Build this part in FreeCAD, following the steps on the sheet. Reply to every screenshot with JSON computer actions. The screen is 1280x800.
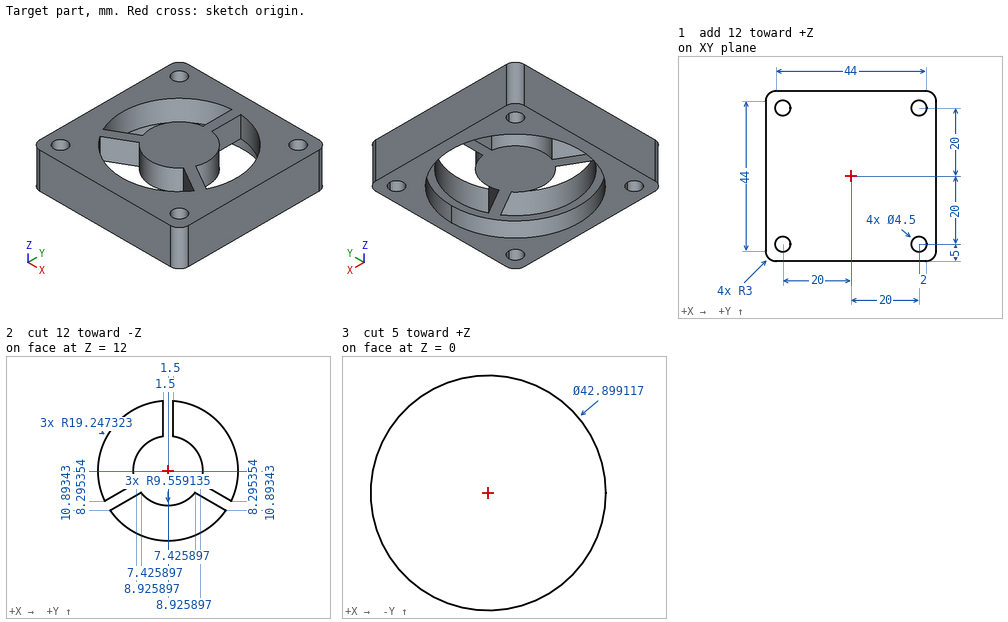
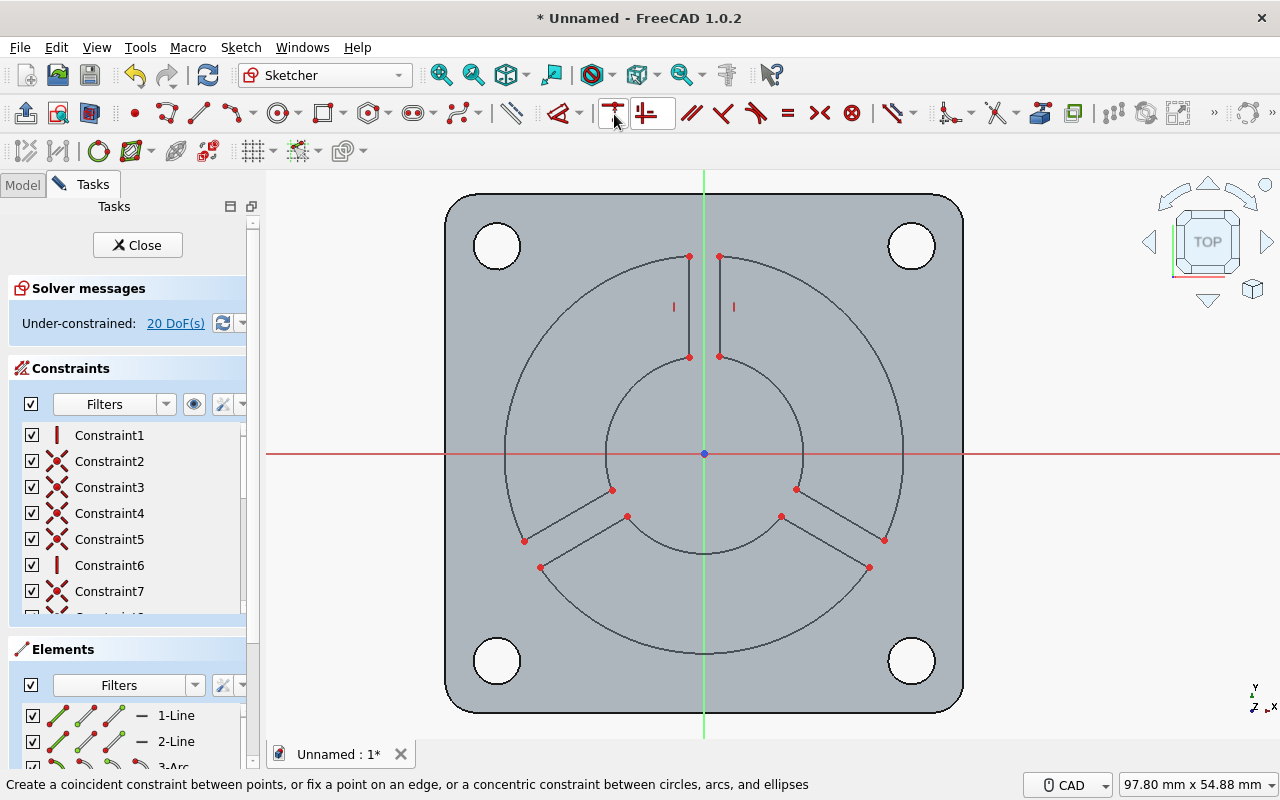
{"action": "left_click", "coordinate": [582, 297]}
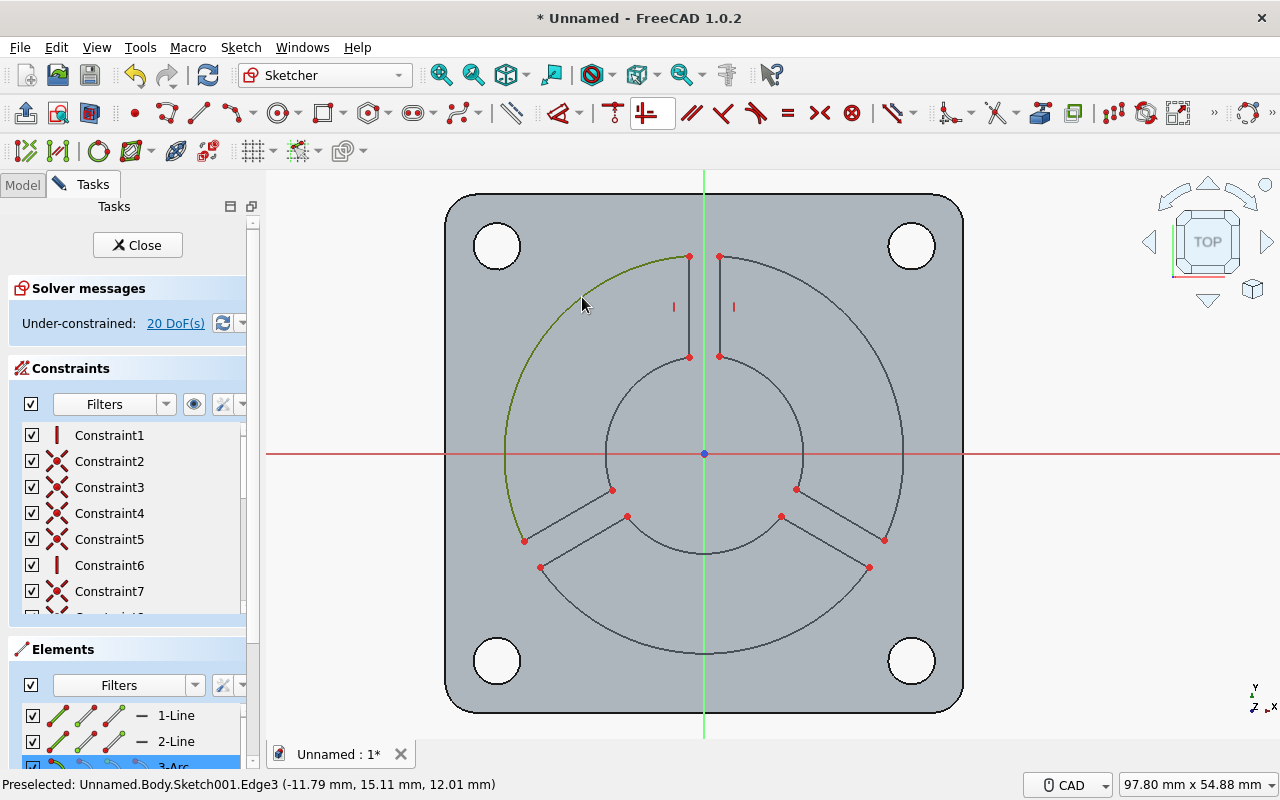
{"action": "left_click", "coordinate": [629, 639]}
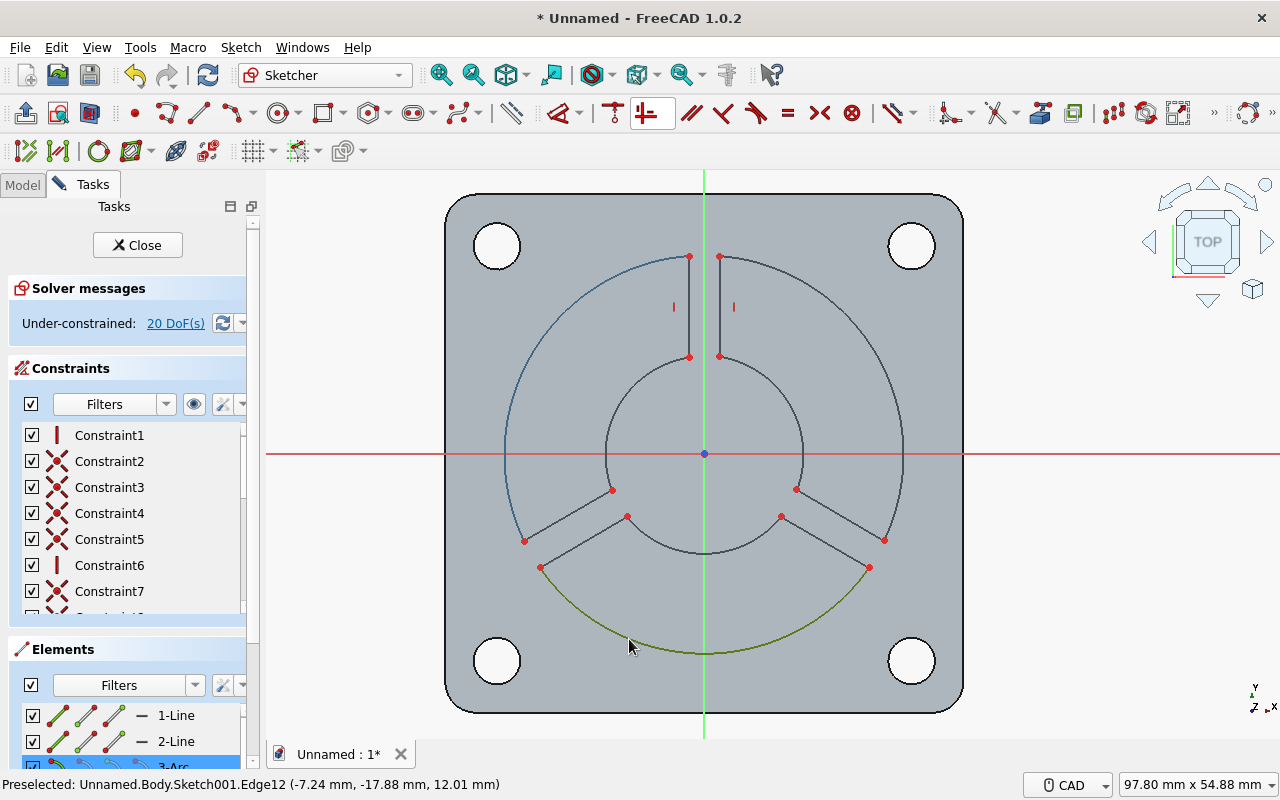
{"action": "left_click", "coordinate": [614, 114]}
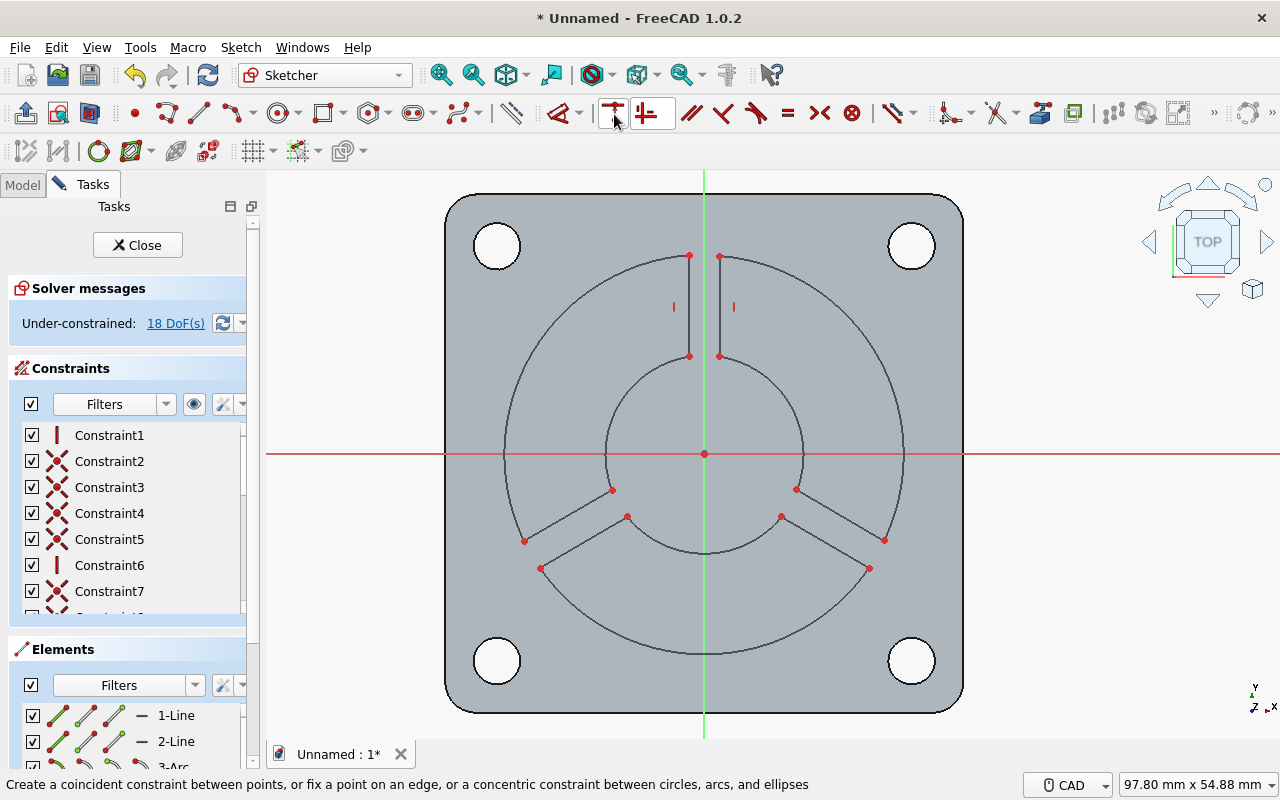
{"action": "left_click_drag", "start_coordinate": [694, 444], "coordinate": [714, 465]}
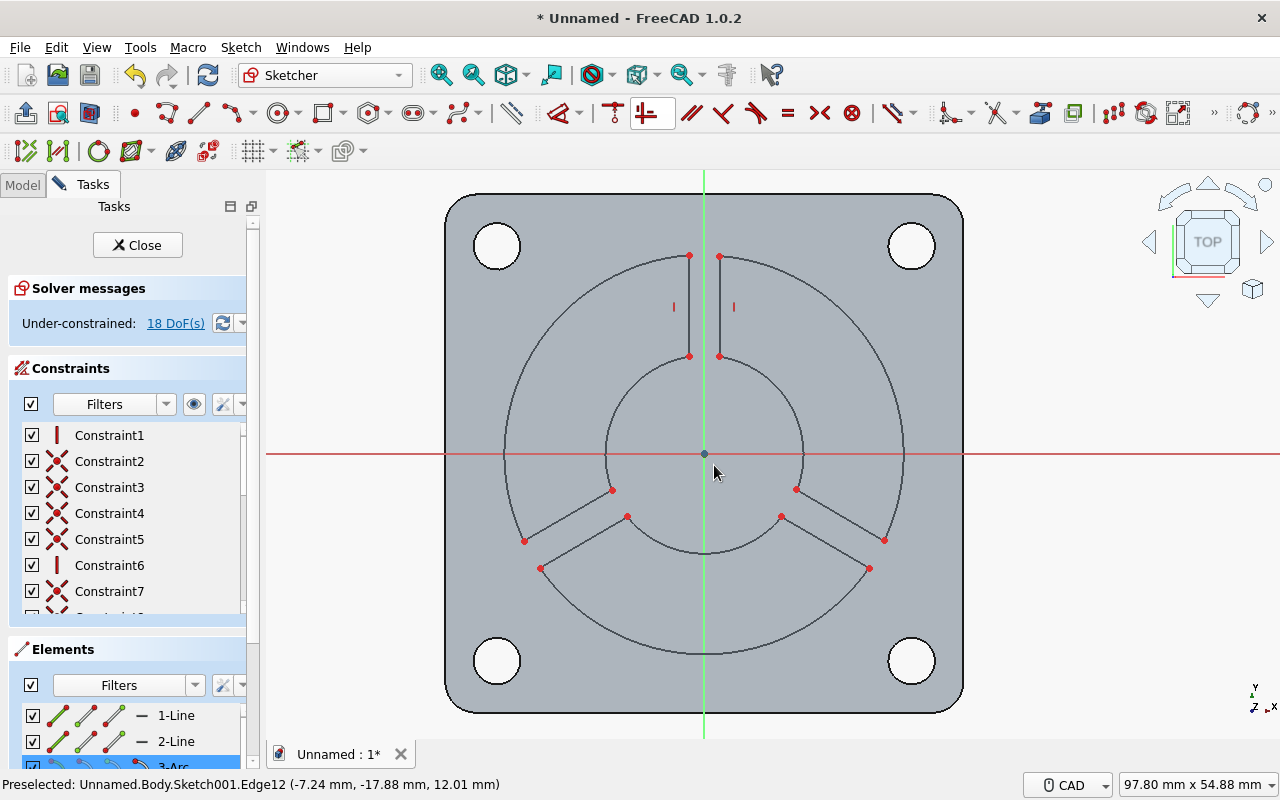
{"action": "left_click", "coordinate": [614, 114]}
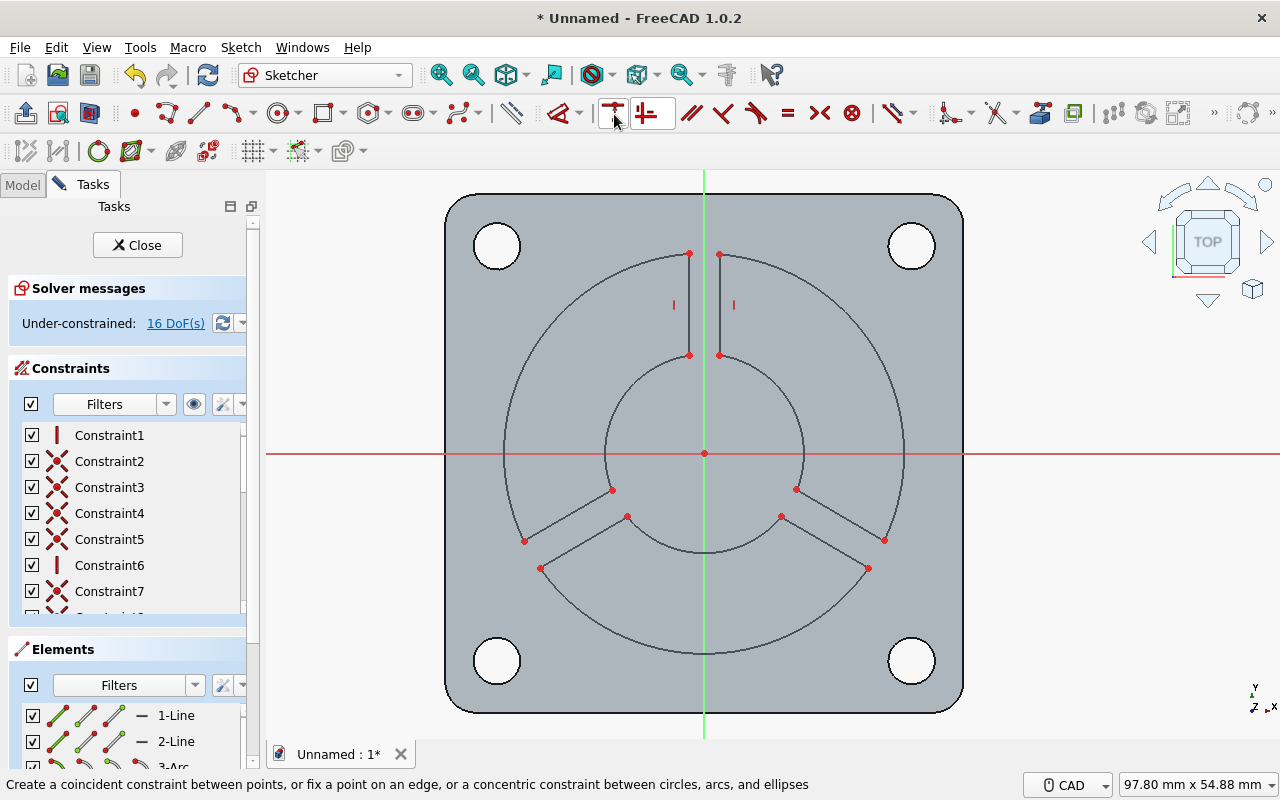
{"action": "left_click", "coordinate": [641, 377]}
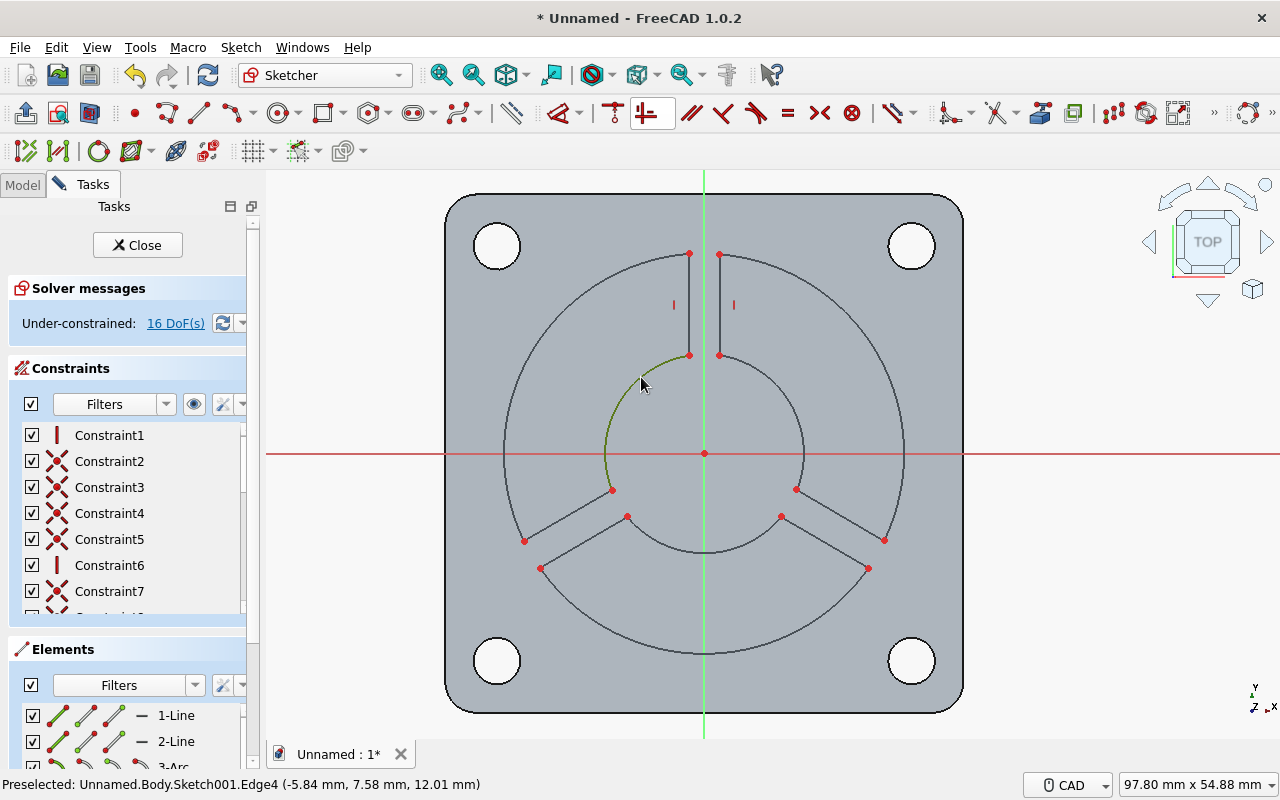
{"action": "left_click", "coordinate": [803, 438]}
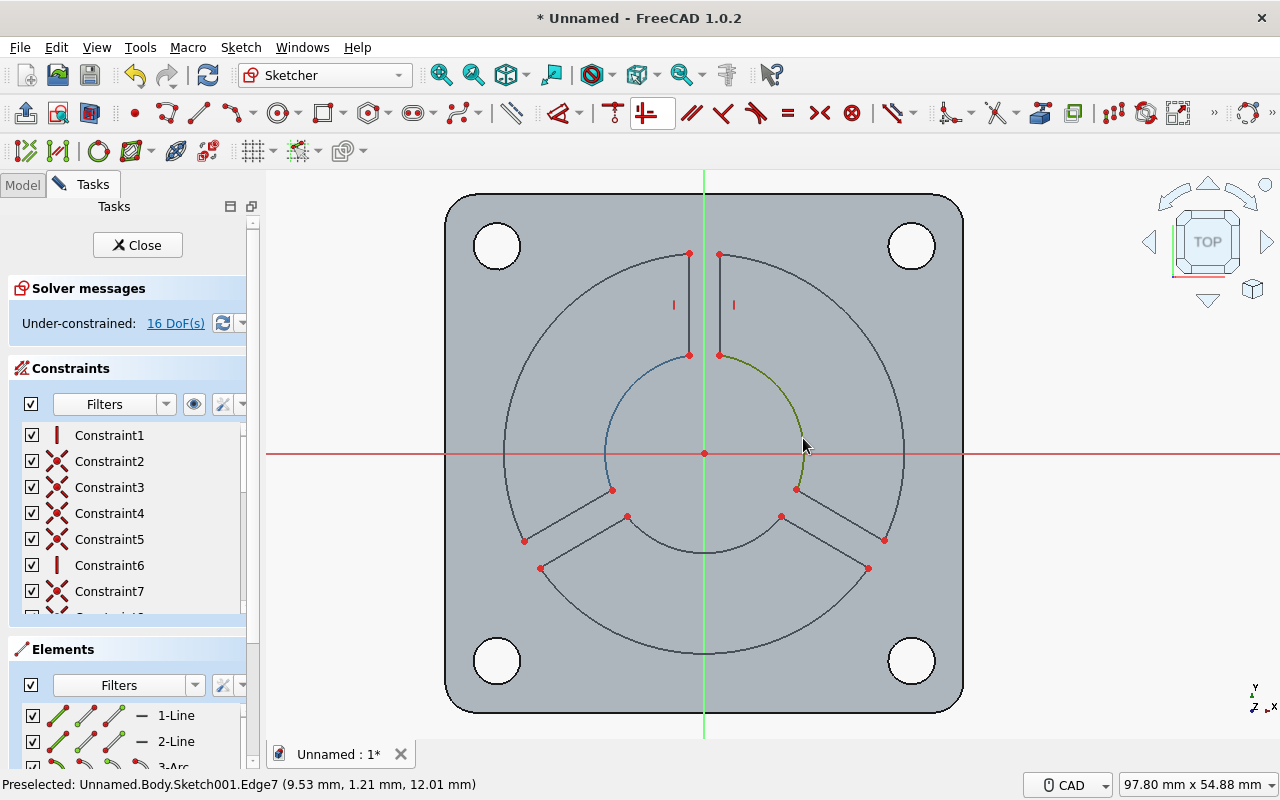
{"action": "left_click", "coordinate": [670, 547]}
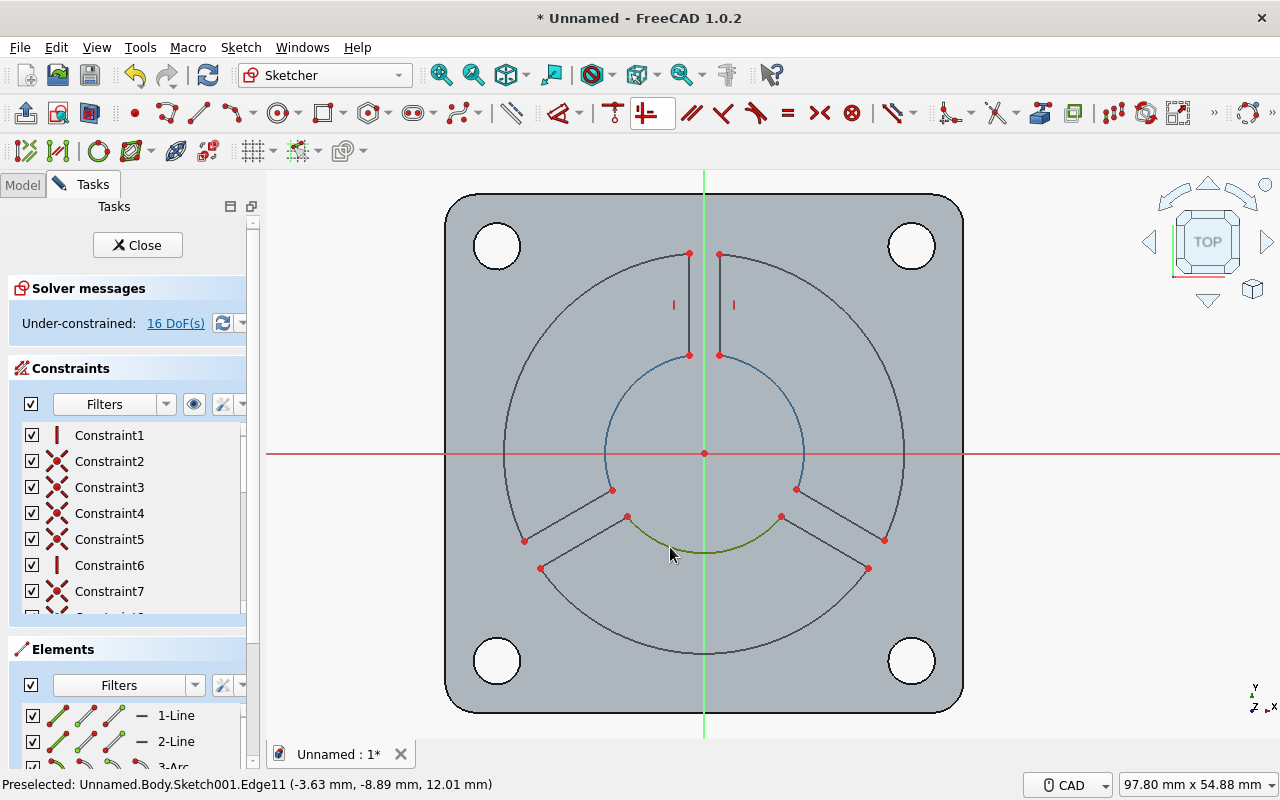
{"action": "left_click", "coordinate": [788, 114]}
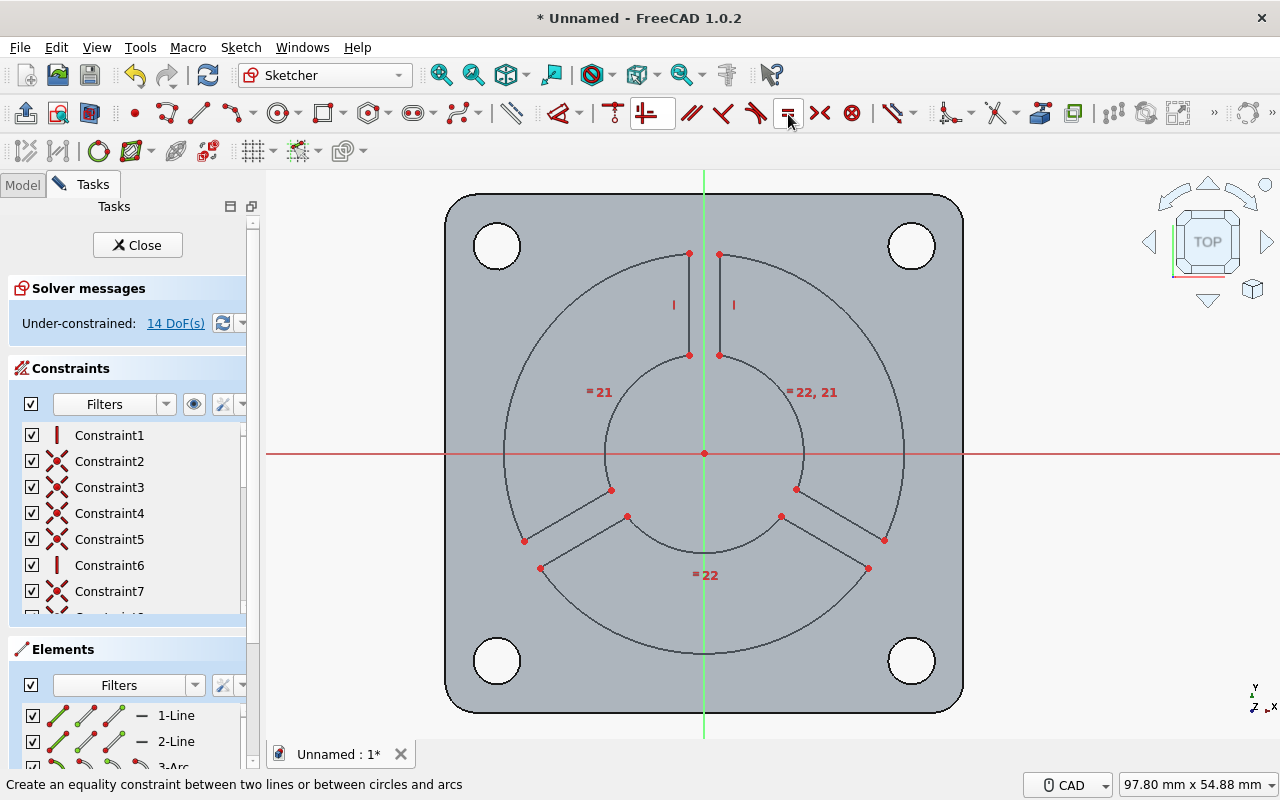
{"action": "left_click", "coordinate": [581, 295]}